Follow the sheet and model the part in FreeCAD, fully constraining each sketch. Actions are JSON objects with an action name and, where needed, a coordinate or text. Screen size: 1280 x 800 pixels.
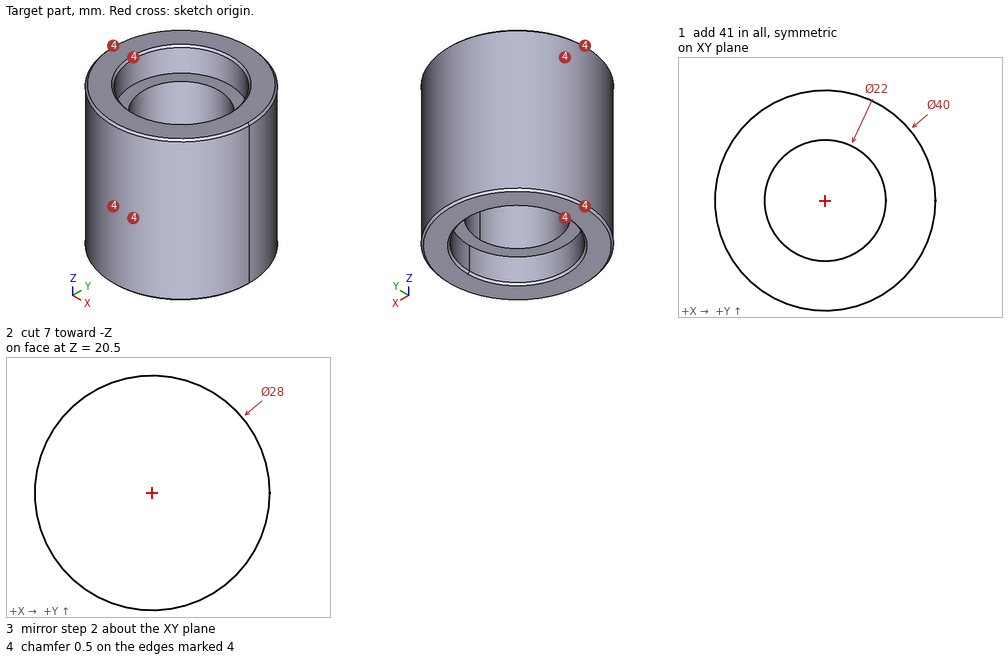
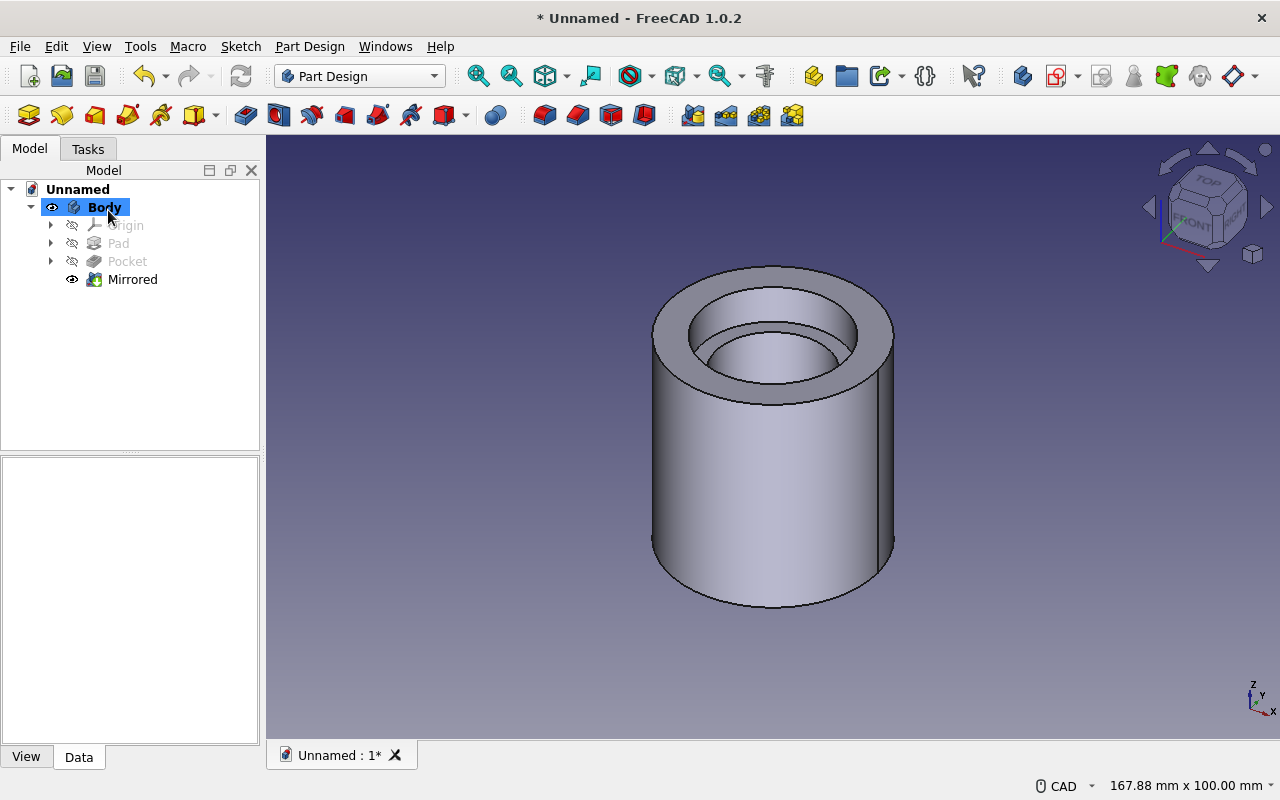
{"action": "left_click", "coordinate": [700, 310]}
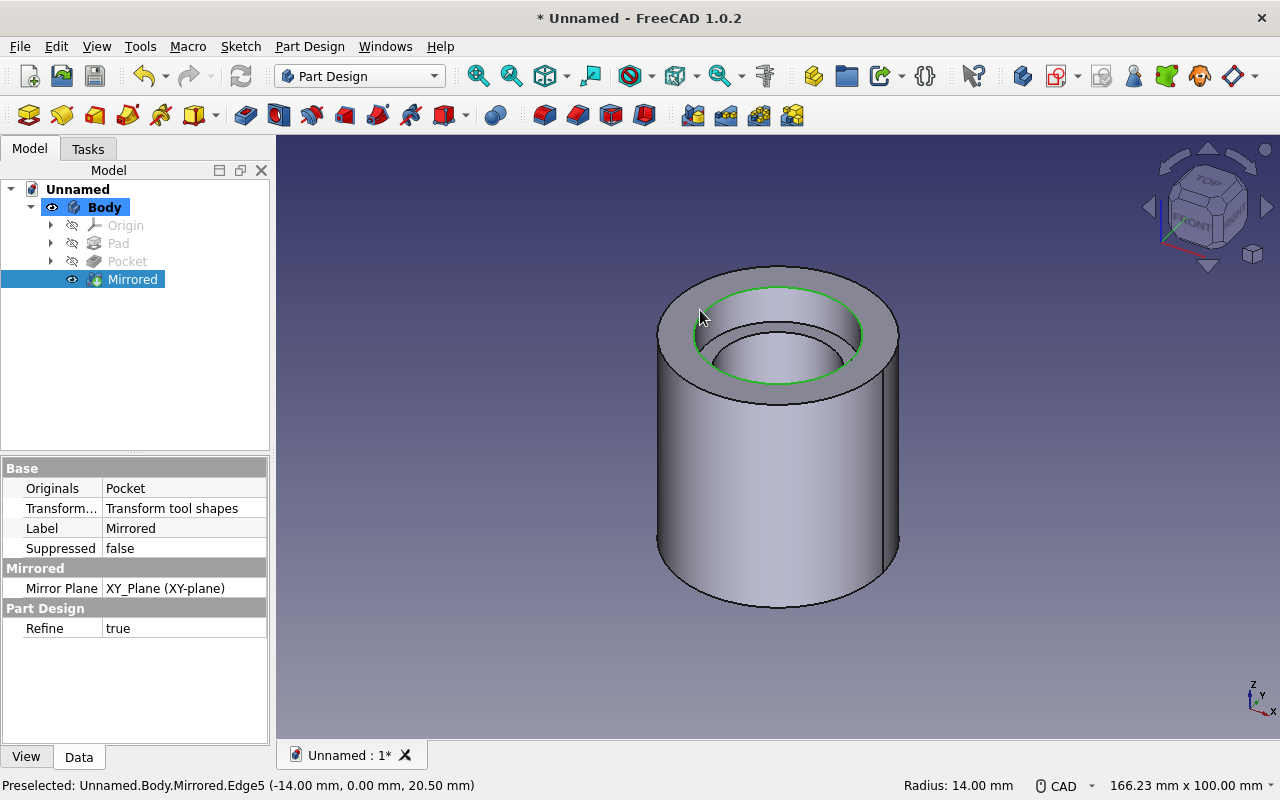
{"action": "left_click", "coordinate": [658, 342], "text": "ctrl"}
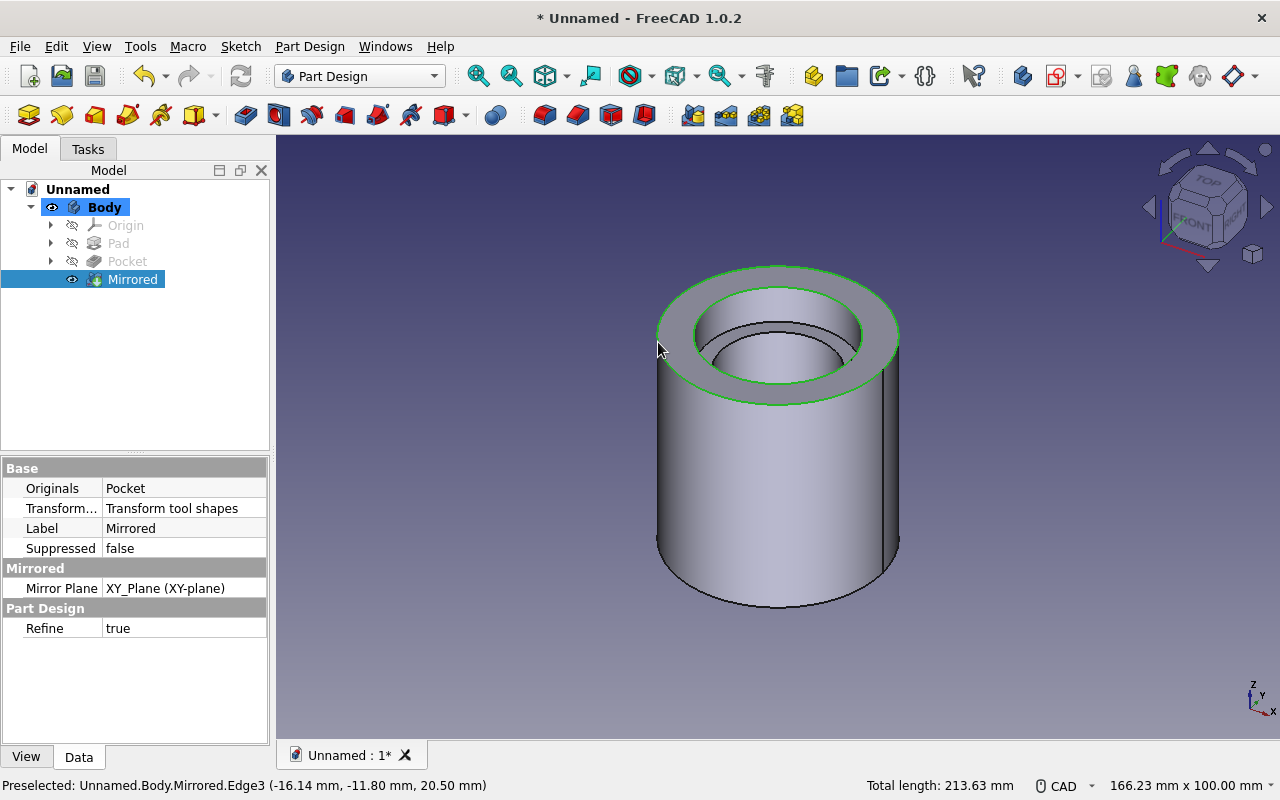
{"action": "key", "text": "0"}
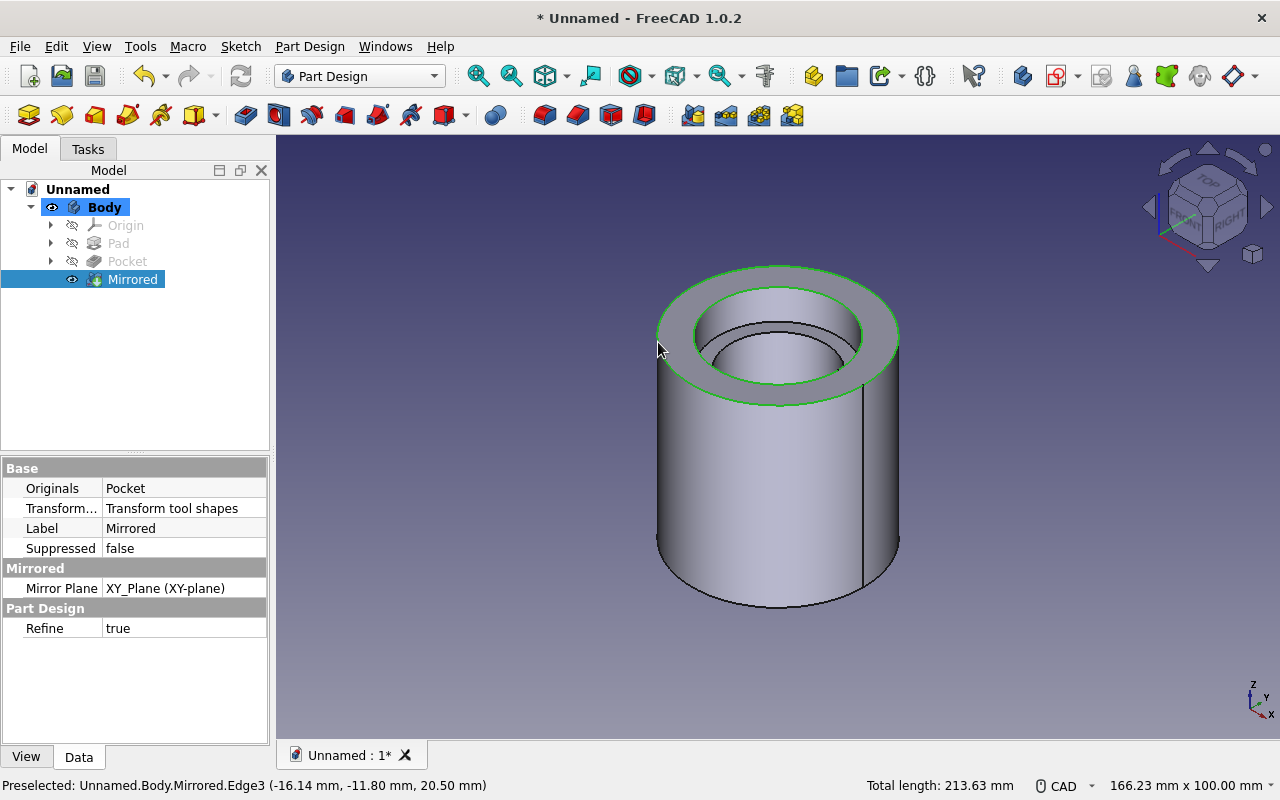
{"action": "key", "text": "2"}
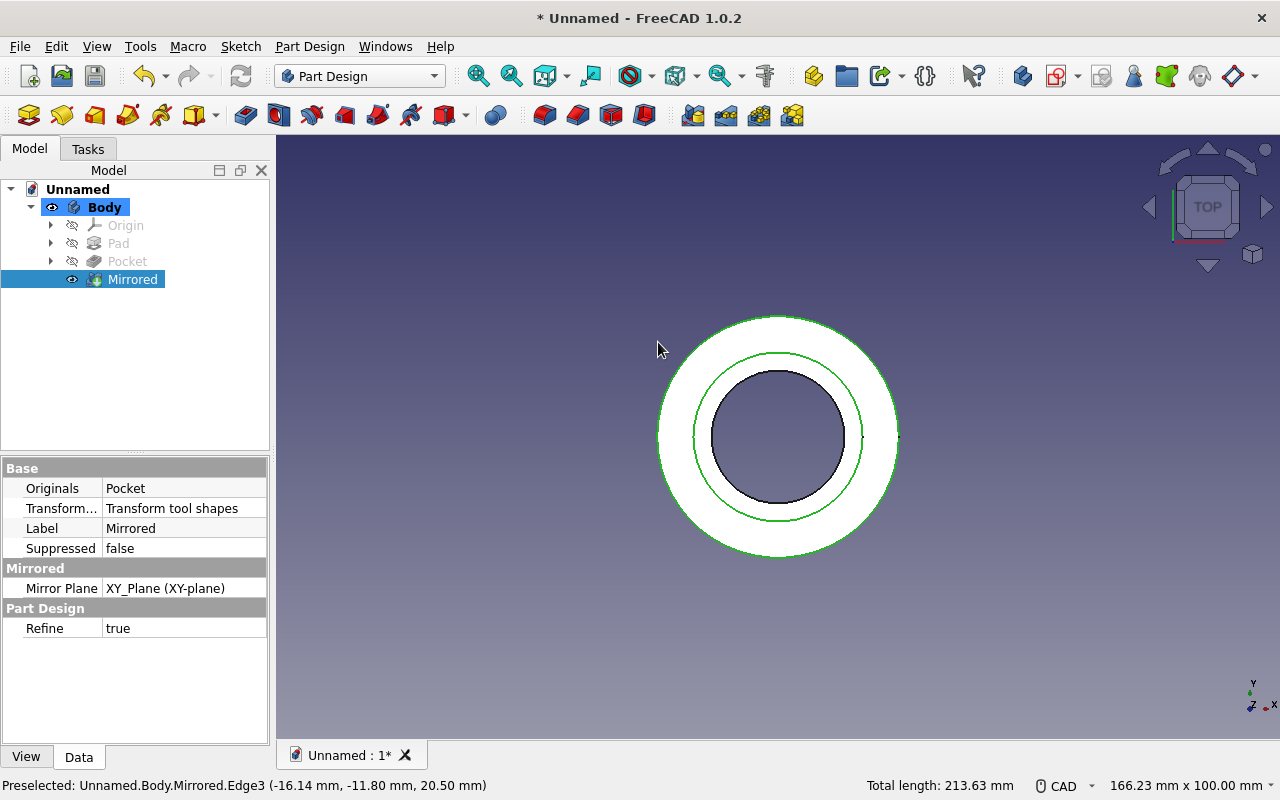
{"action": "left_click", "coordinate": [479, 76]}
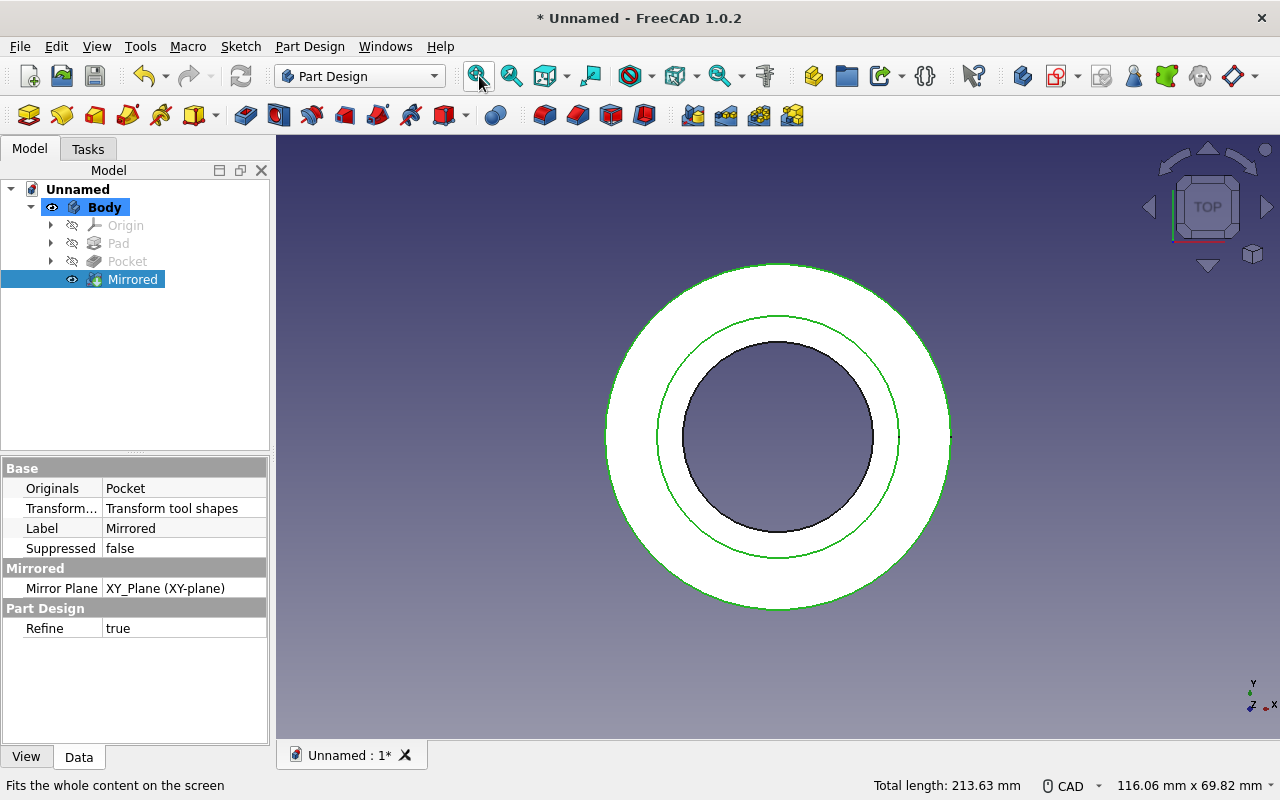
{"action": "key", "text": "1"}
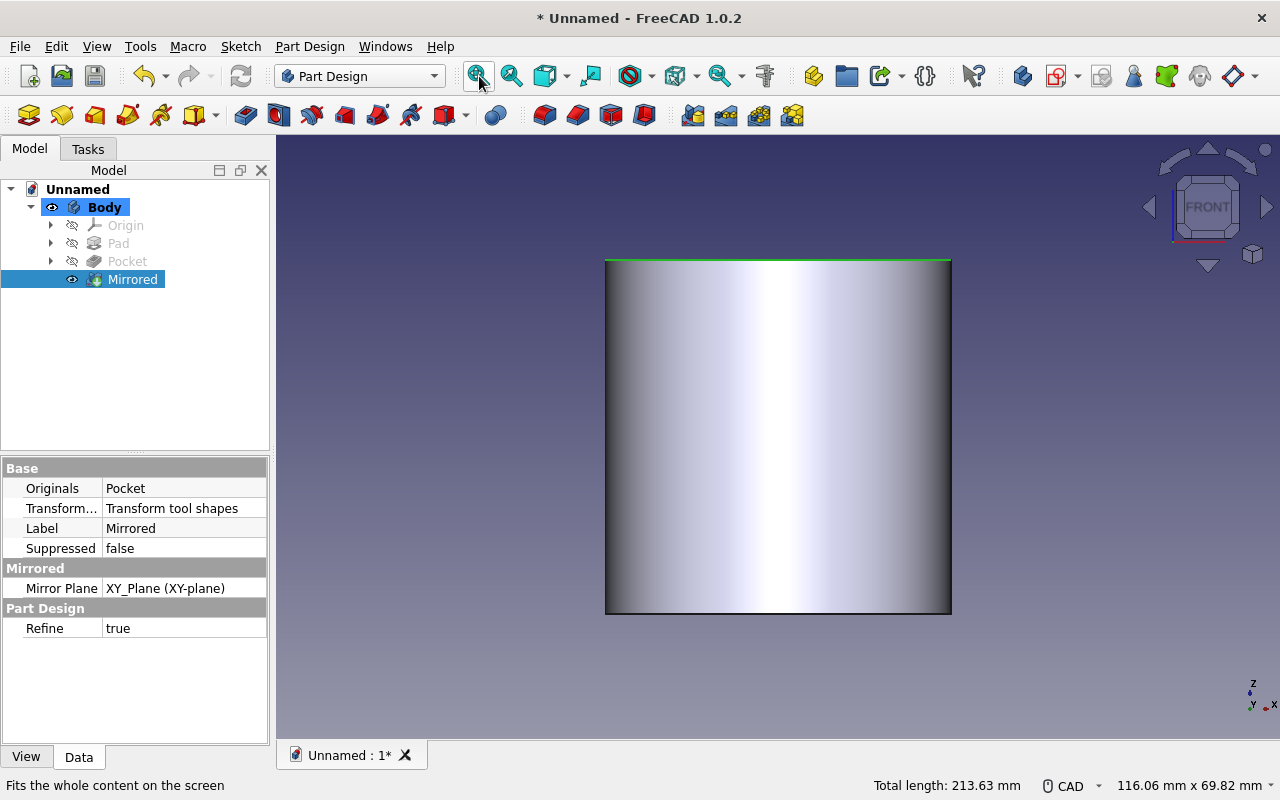
{"action": "left_click", "coordinate": [638, 613], "text": "ctrl"}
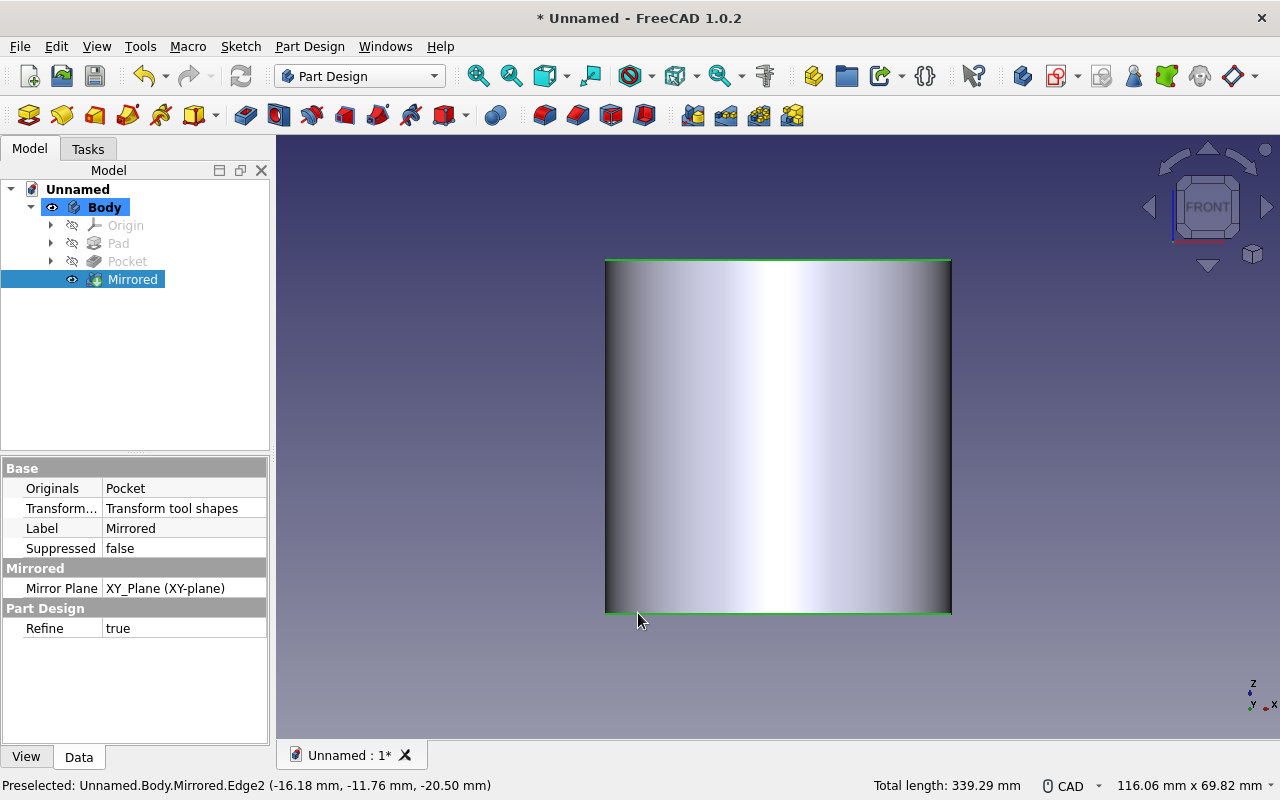
{"action": "key", "text": "3"}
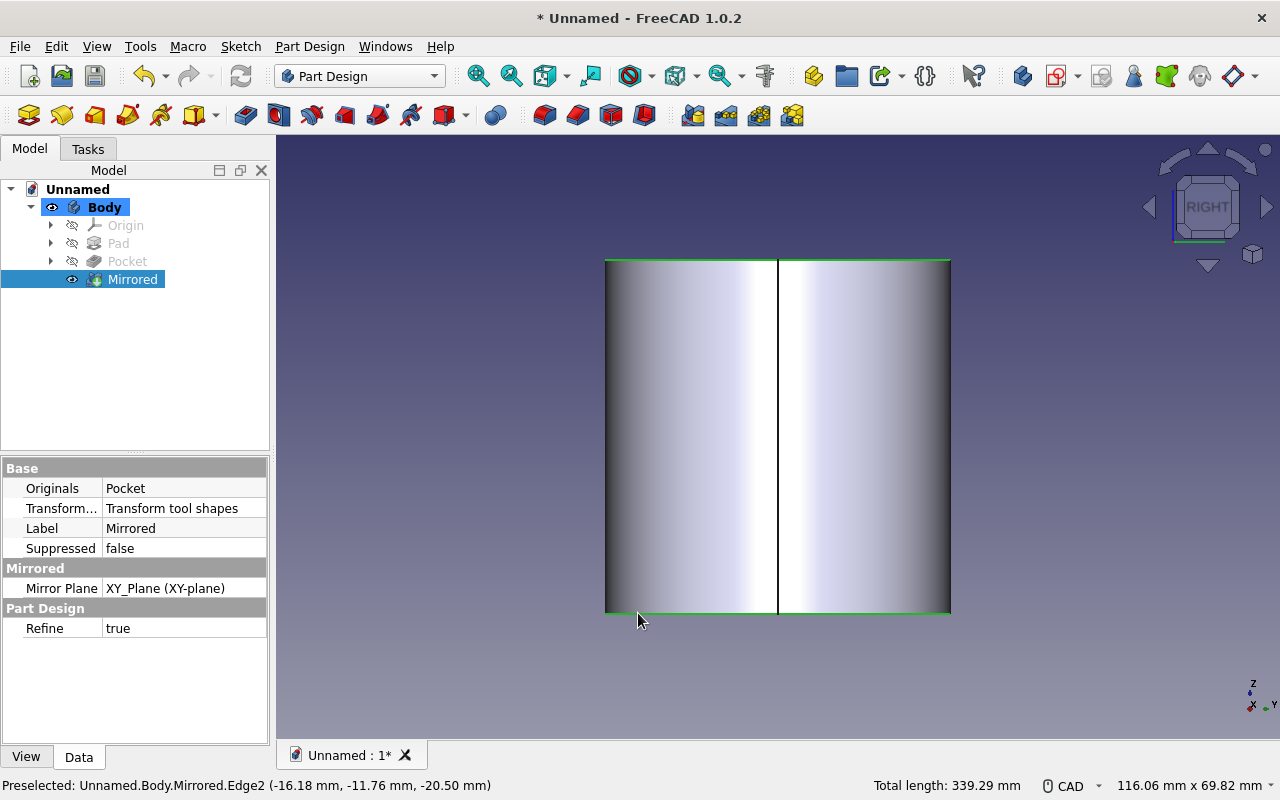
{"action": "key", "text": "5"}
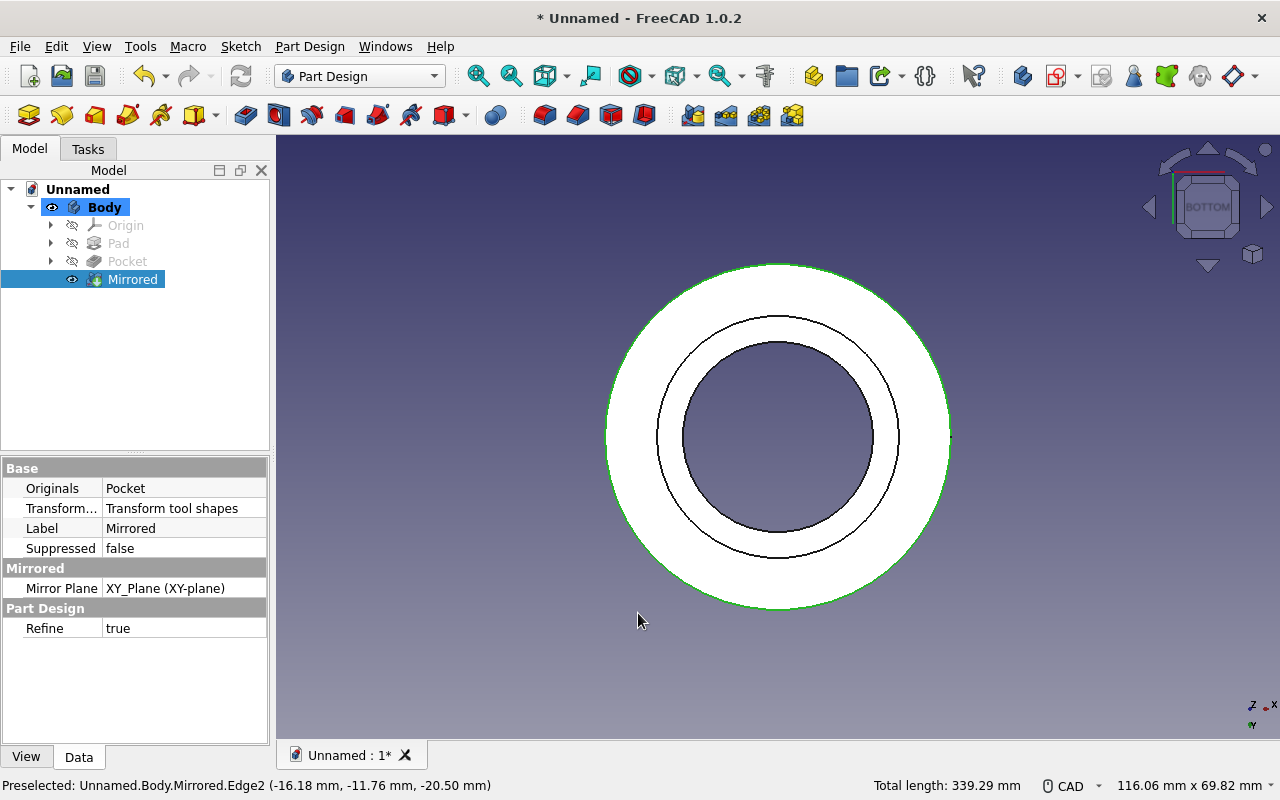
{"action": "left_click", "coordinate": [657, 436], "text": "ctrl"}